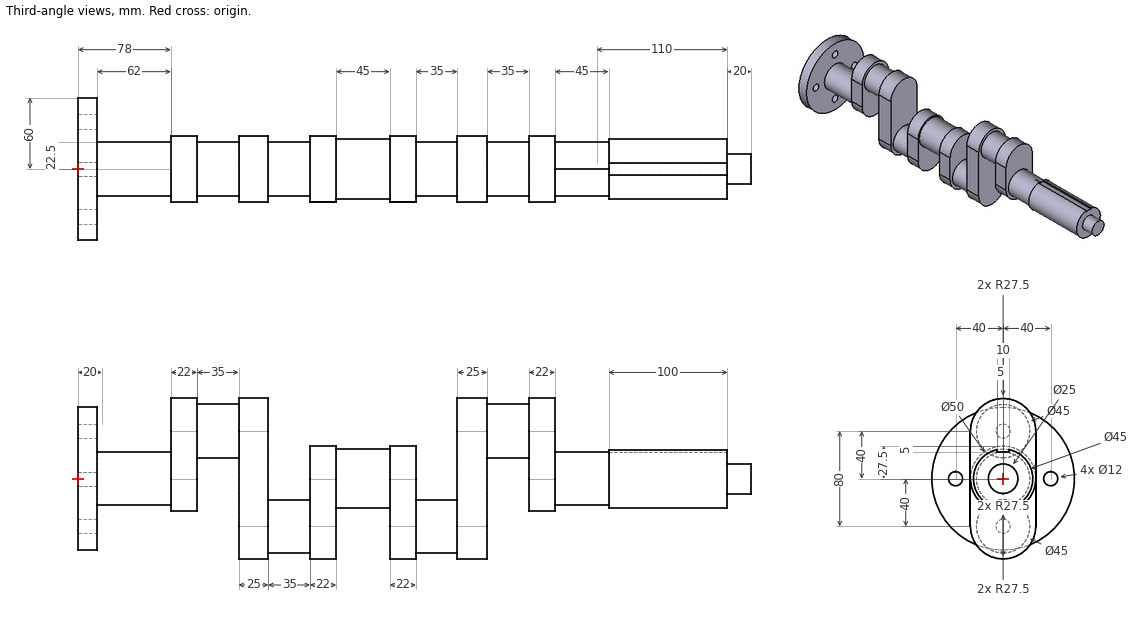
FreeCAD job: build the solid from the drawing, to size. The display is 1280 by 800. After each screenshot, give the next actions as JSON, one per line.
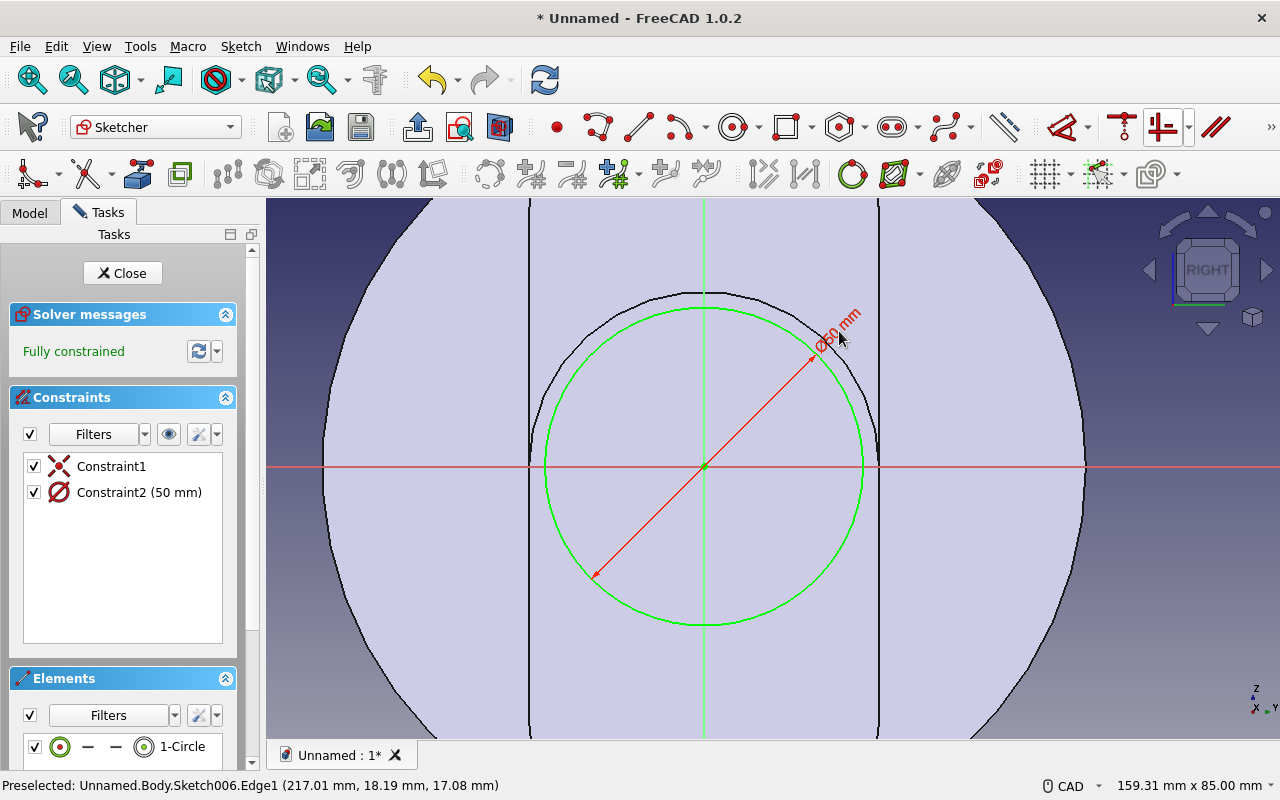
{"action": "left_click", "coordinate": [123, 273]}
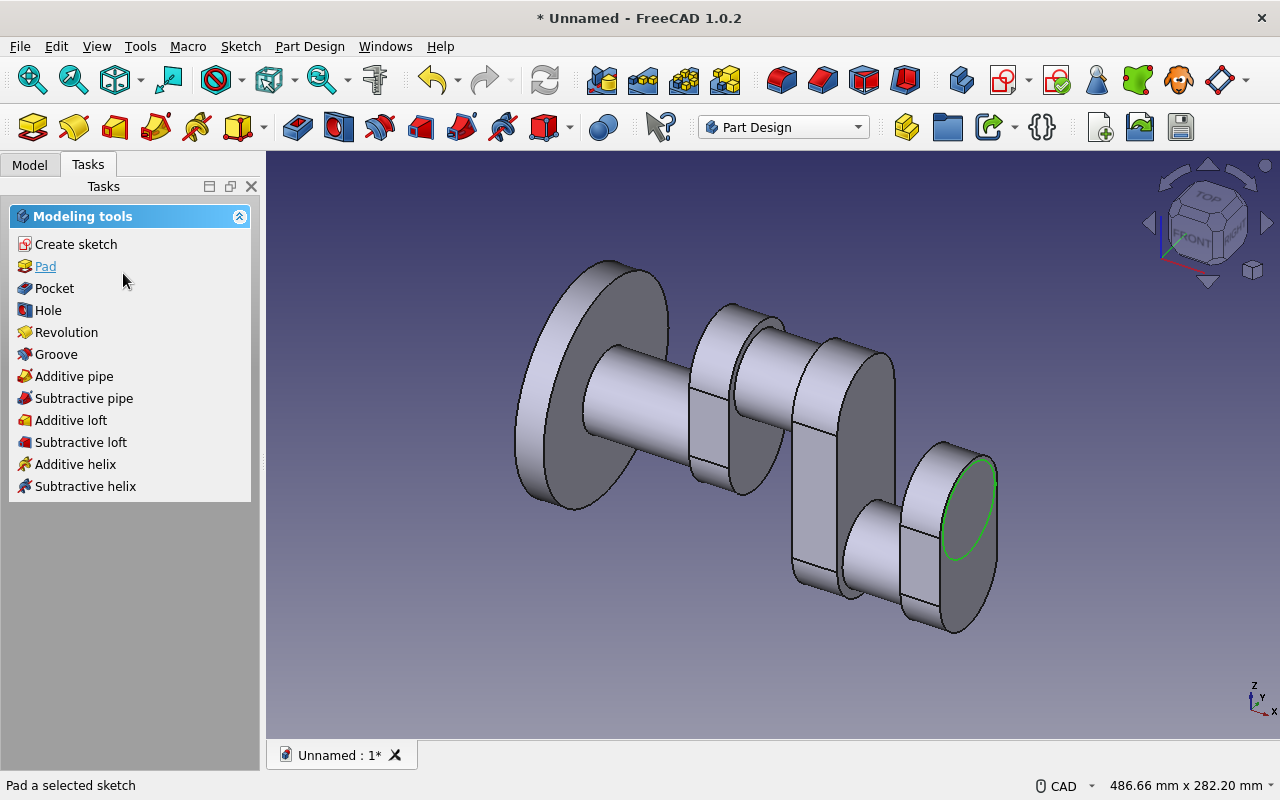
{"action": "left_click", "coordinate": [33, 128]}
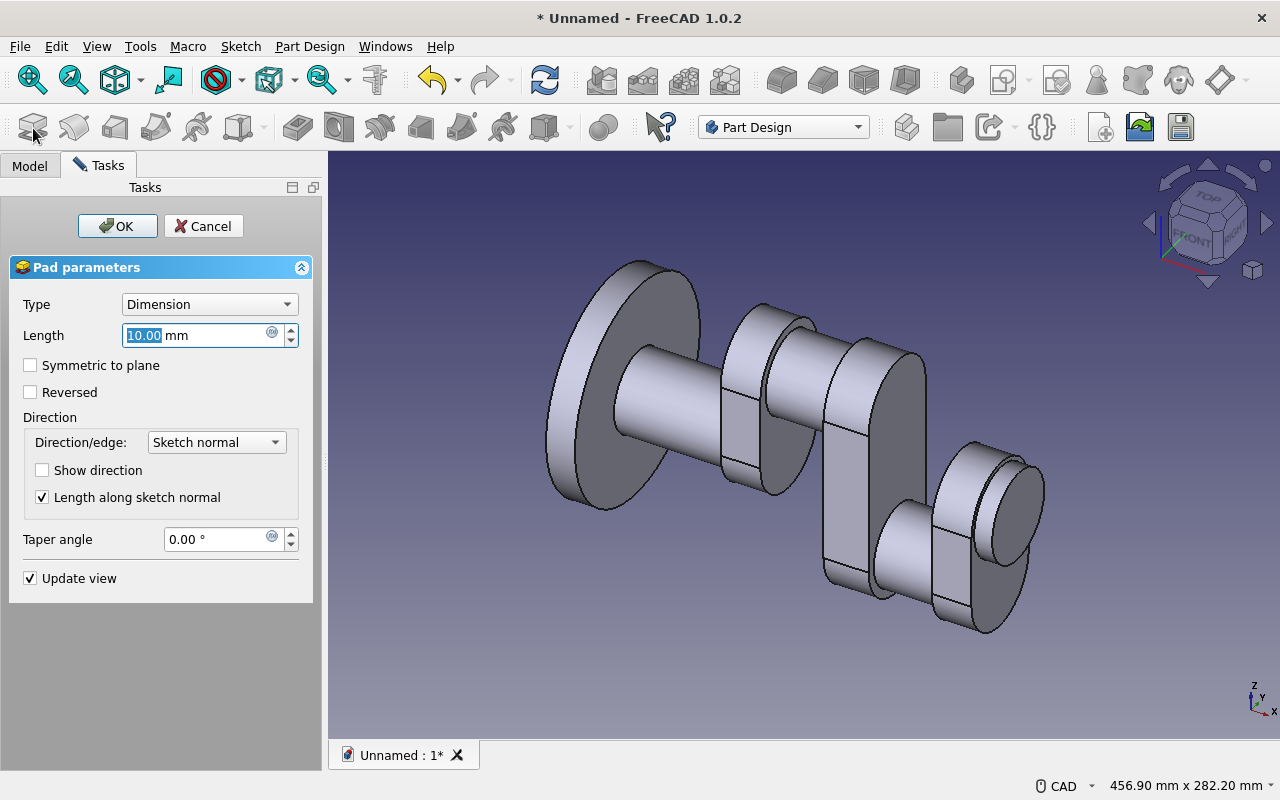
{"action": "type", "text": "45"}
{"action": "key", "text": "Tab"}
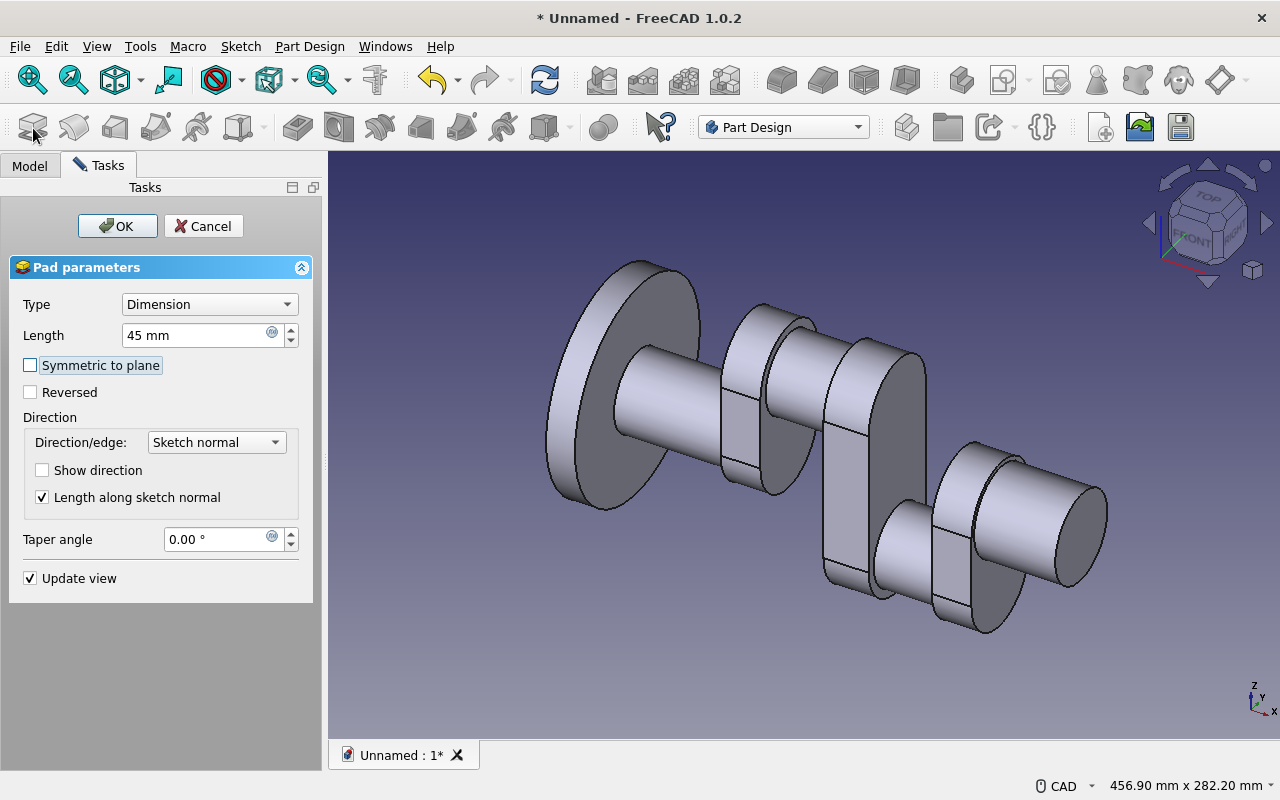
{"action": "left_click", "coordinate": [118, 226]}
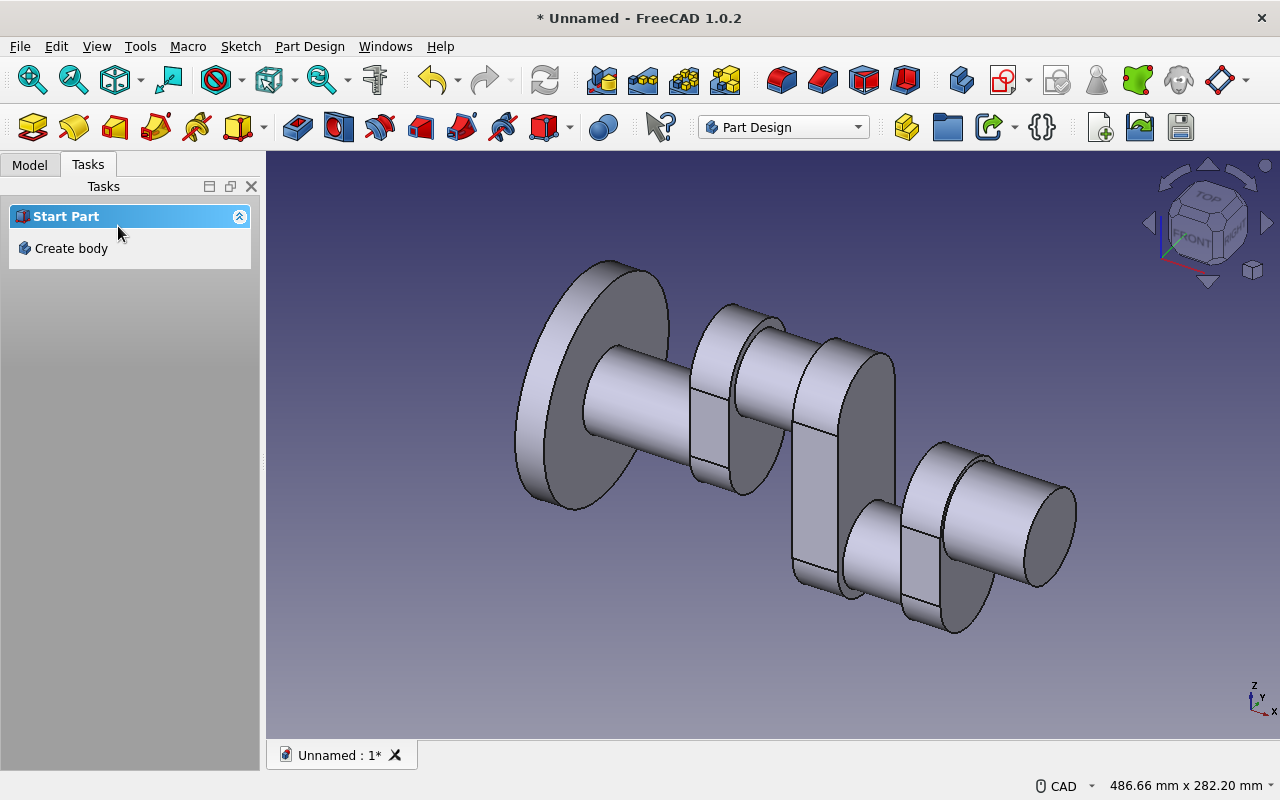
{"action": "left_click", "coordinate": [1050, 536]}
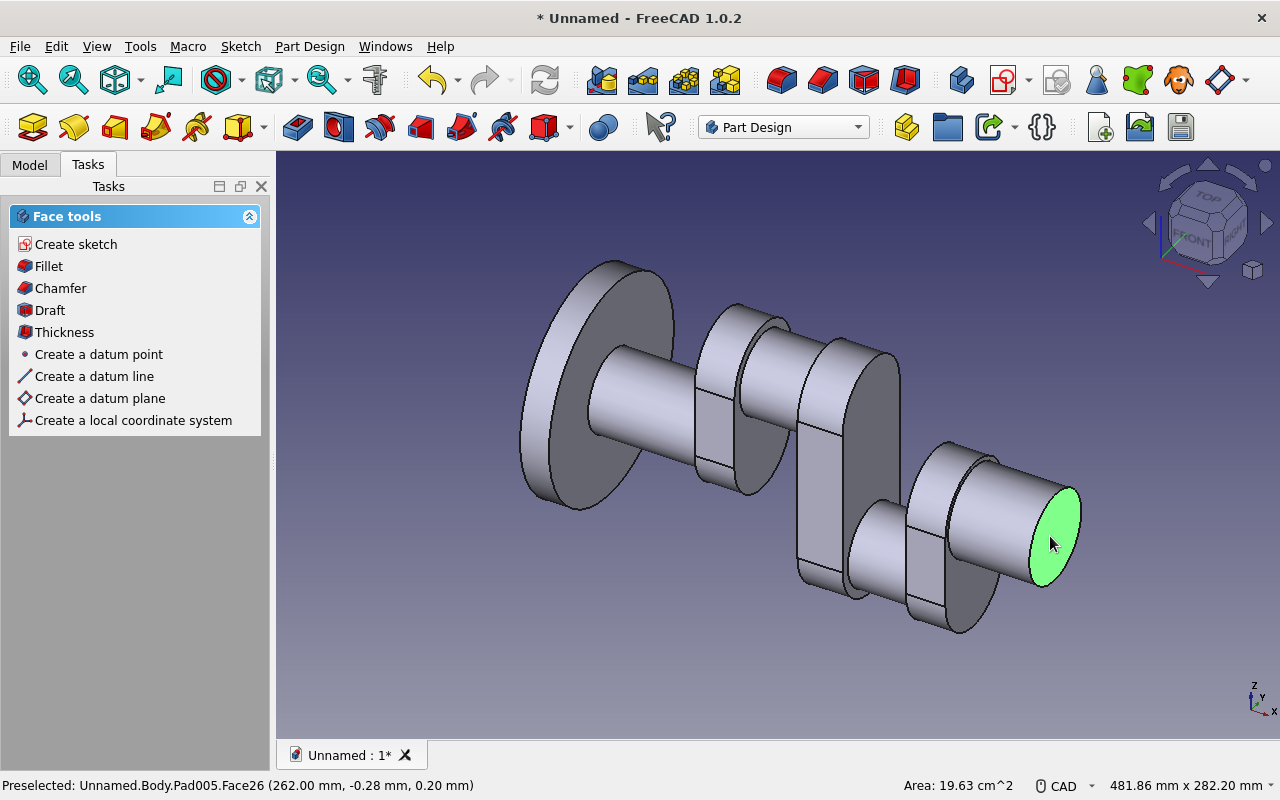
{"action": "left_click", "coordinate": [1002, 80]}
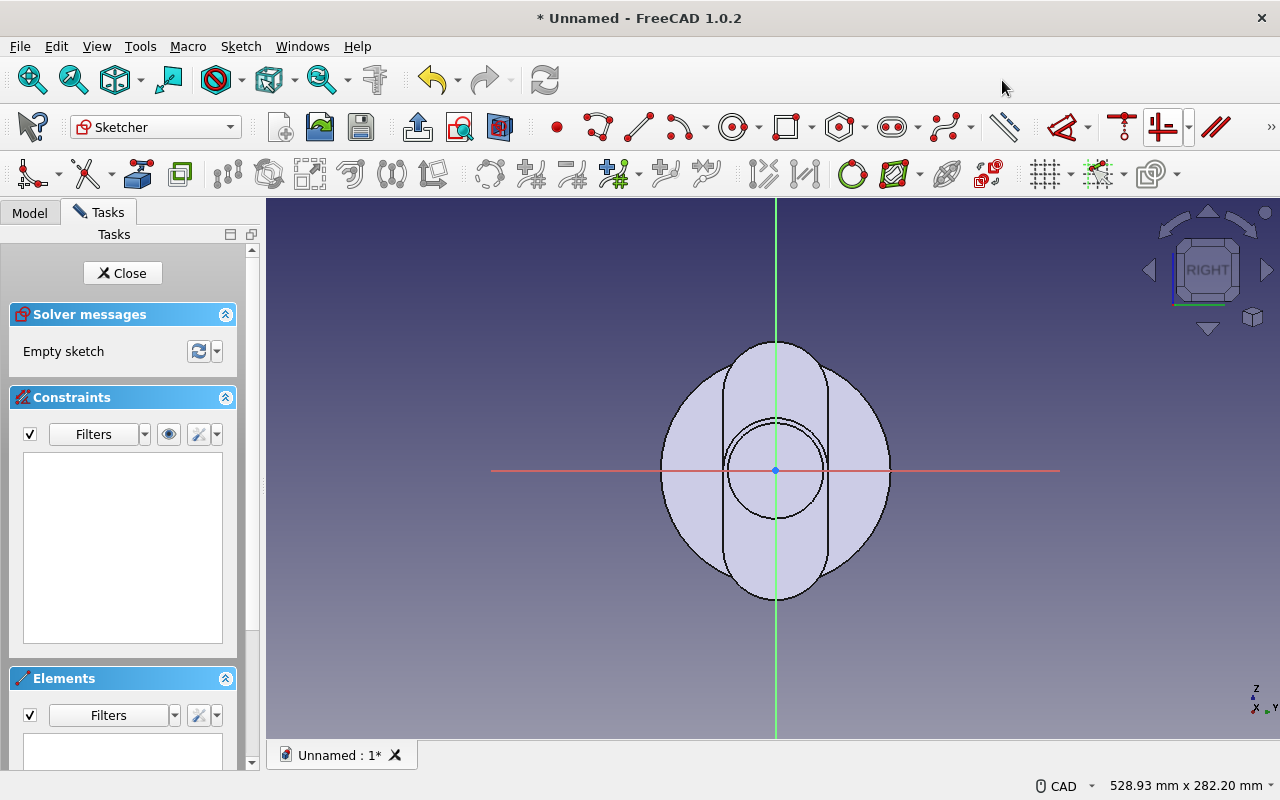
{"action": "scroll", "coordinate": [862, 559], "scroll_direction": "up", "scroll_amount": 3}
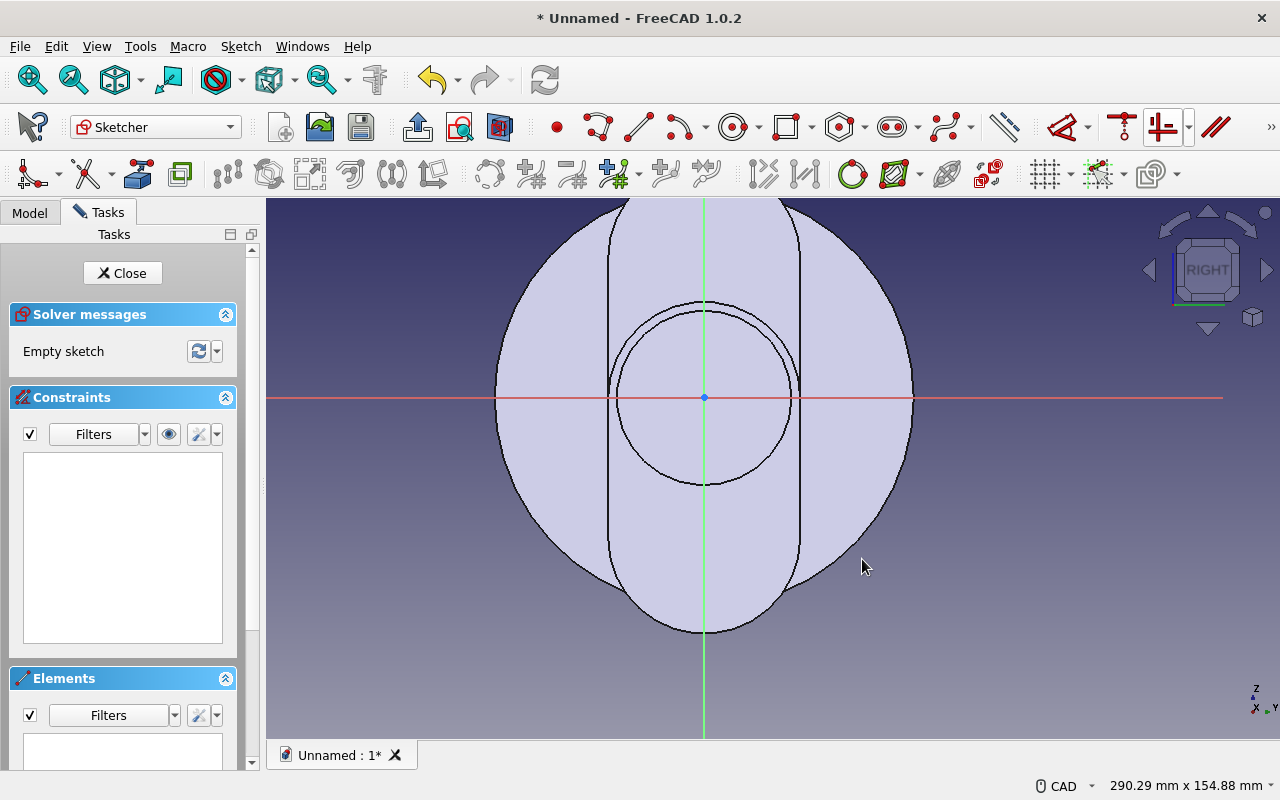
{"action": "left_click", "coordinate": [892, 128]}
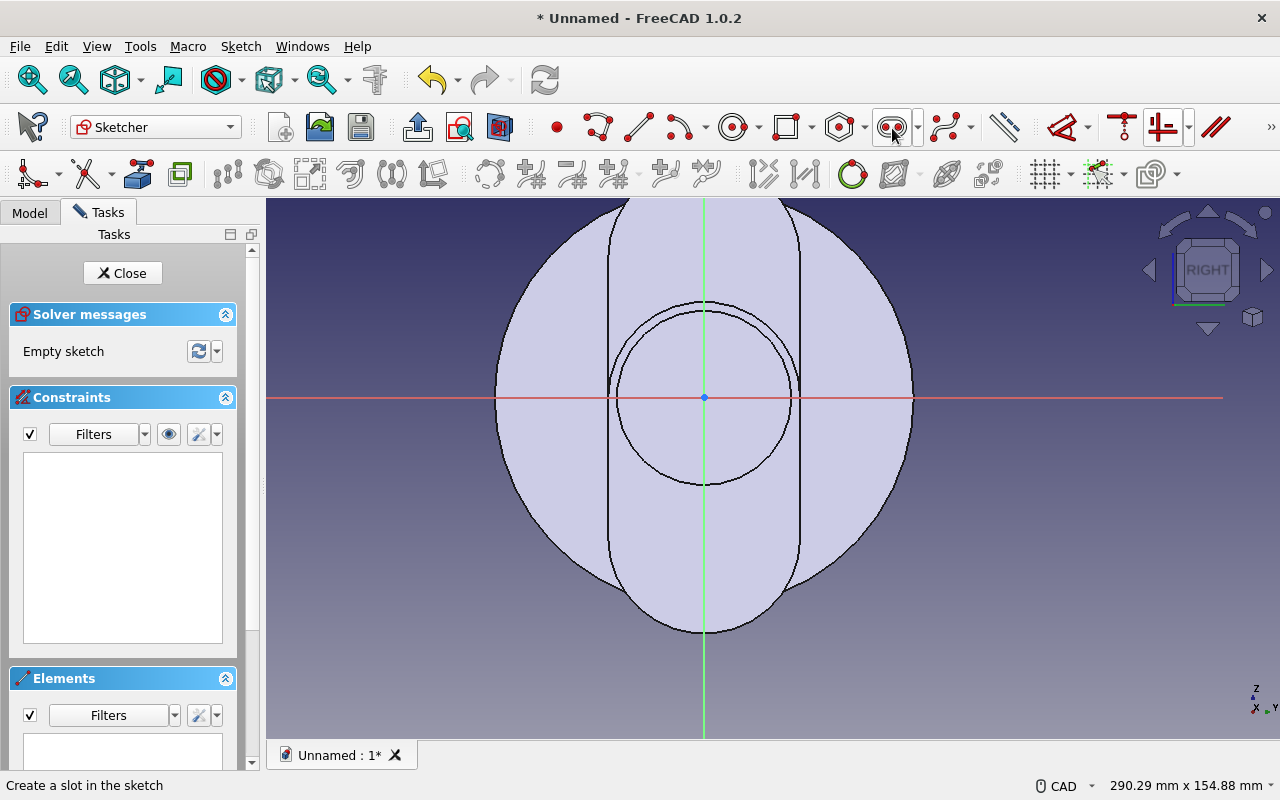
{"action": "left_click", "coordinate": [704, 398]}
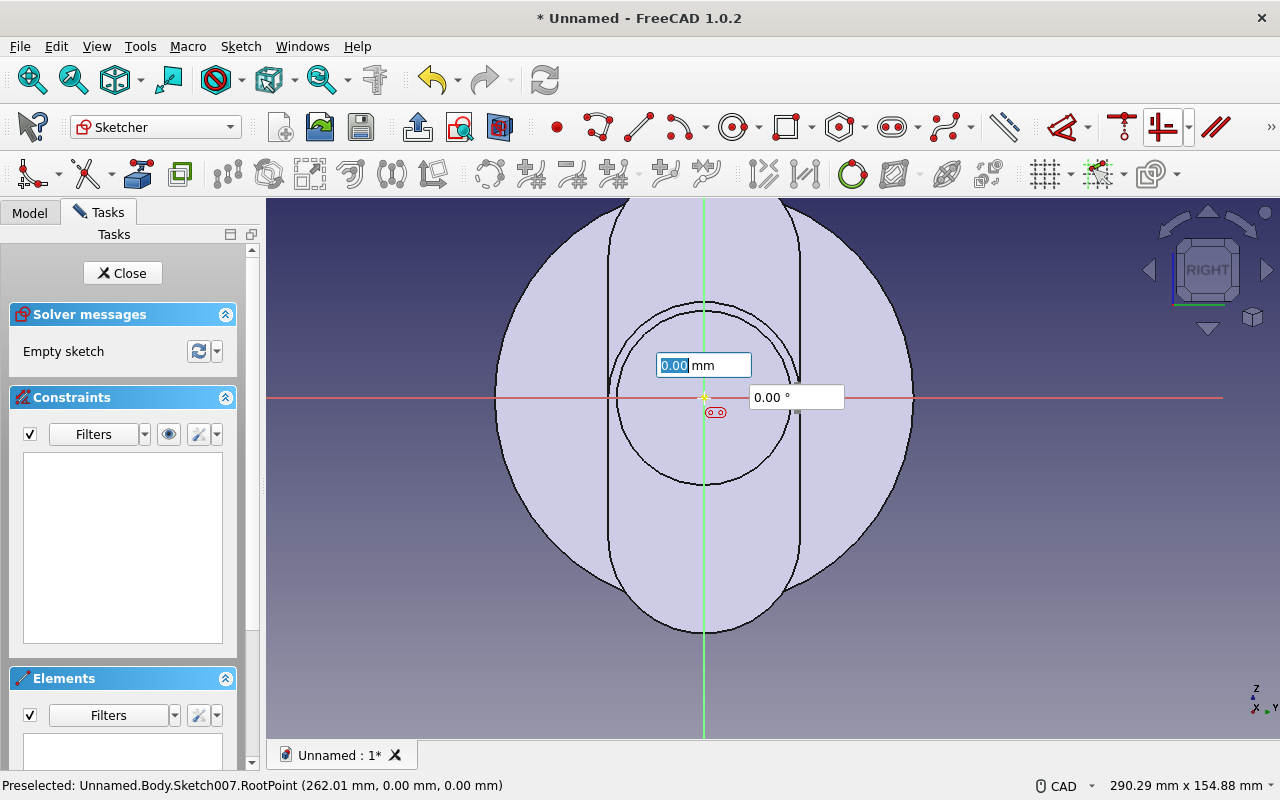
{"action": "left_click", "coordinate": [713, 538]}